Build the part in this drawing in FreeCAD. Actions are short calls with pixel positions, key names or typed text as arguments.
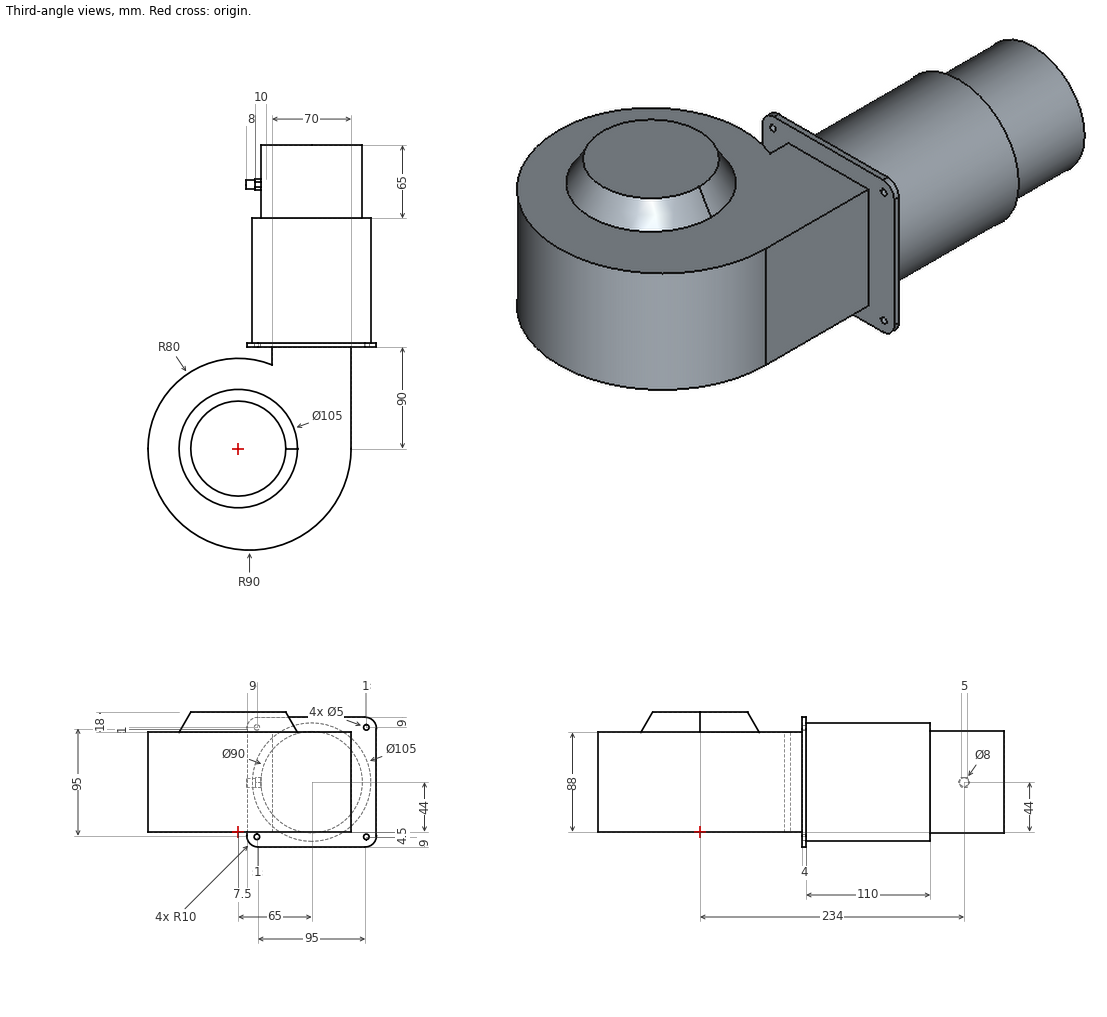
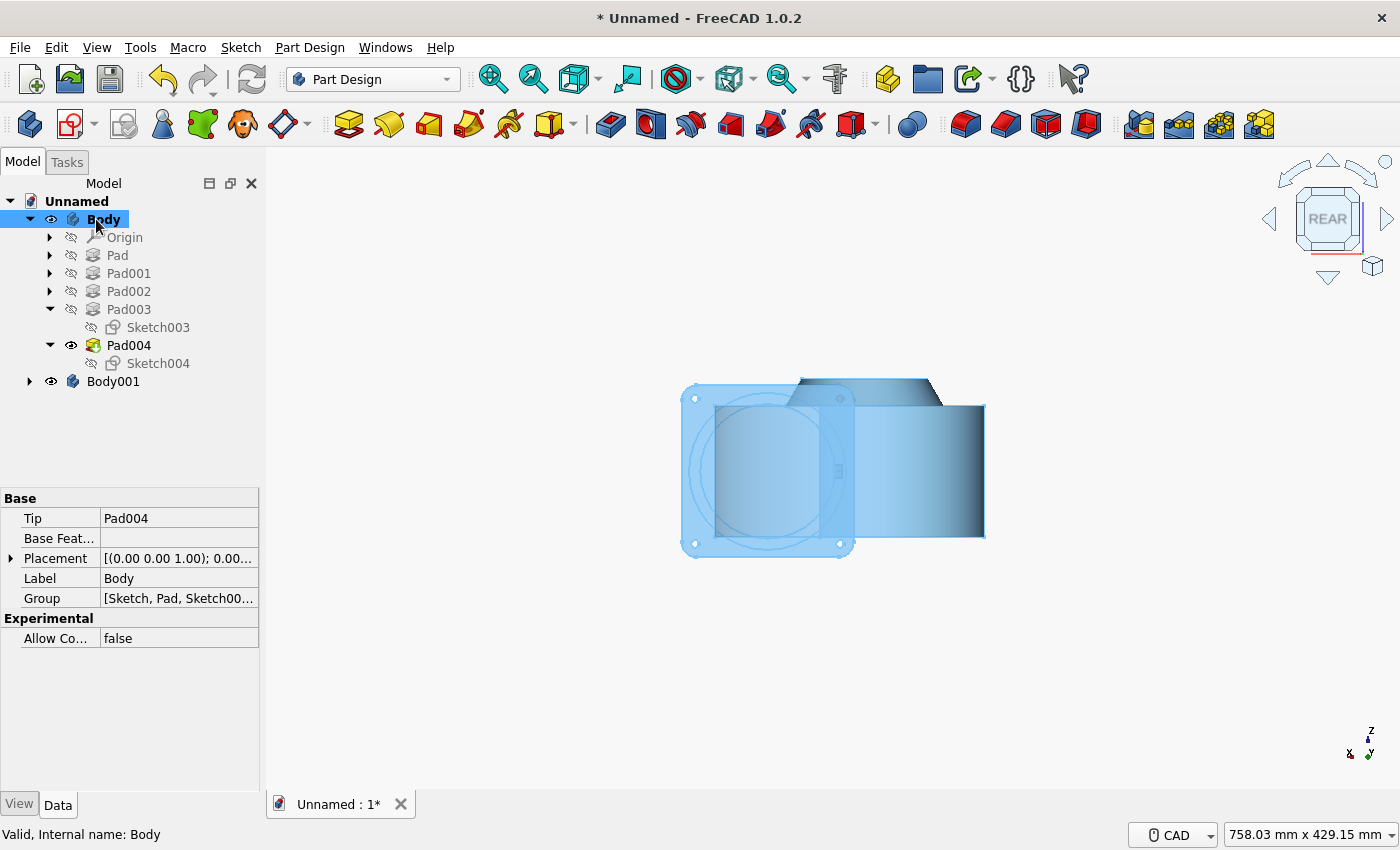
click(96, 381)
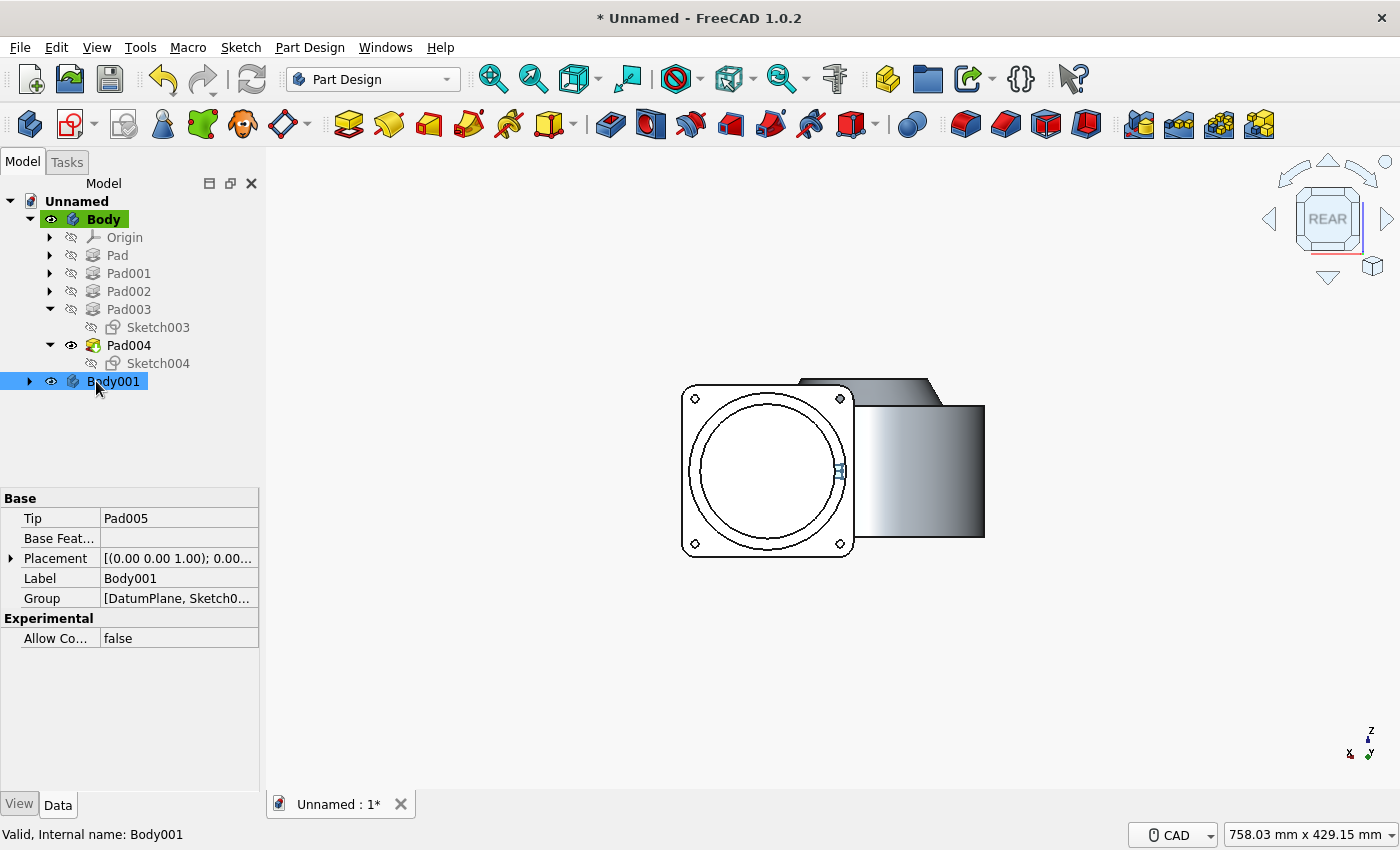
click(914, 124)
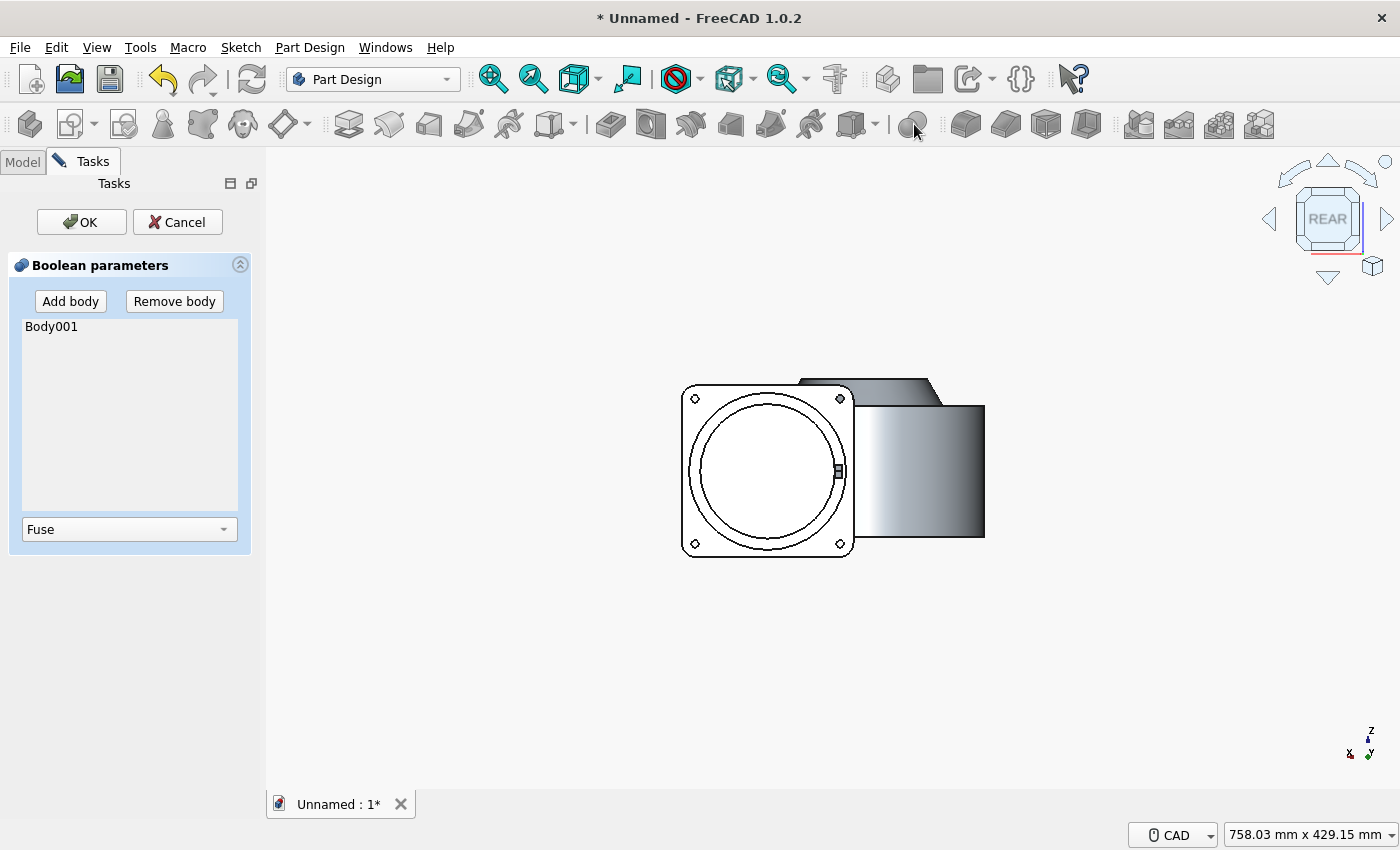
click(82, 222)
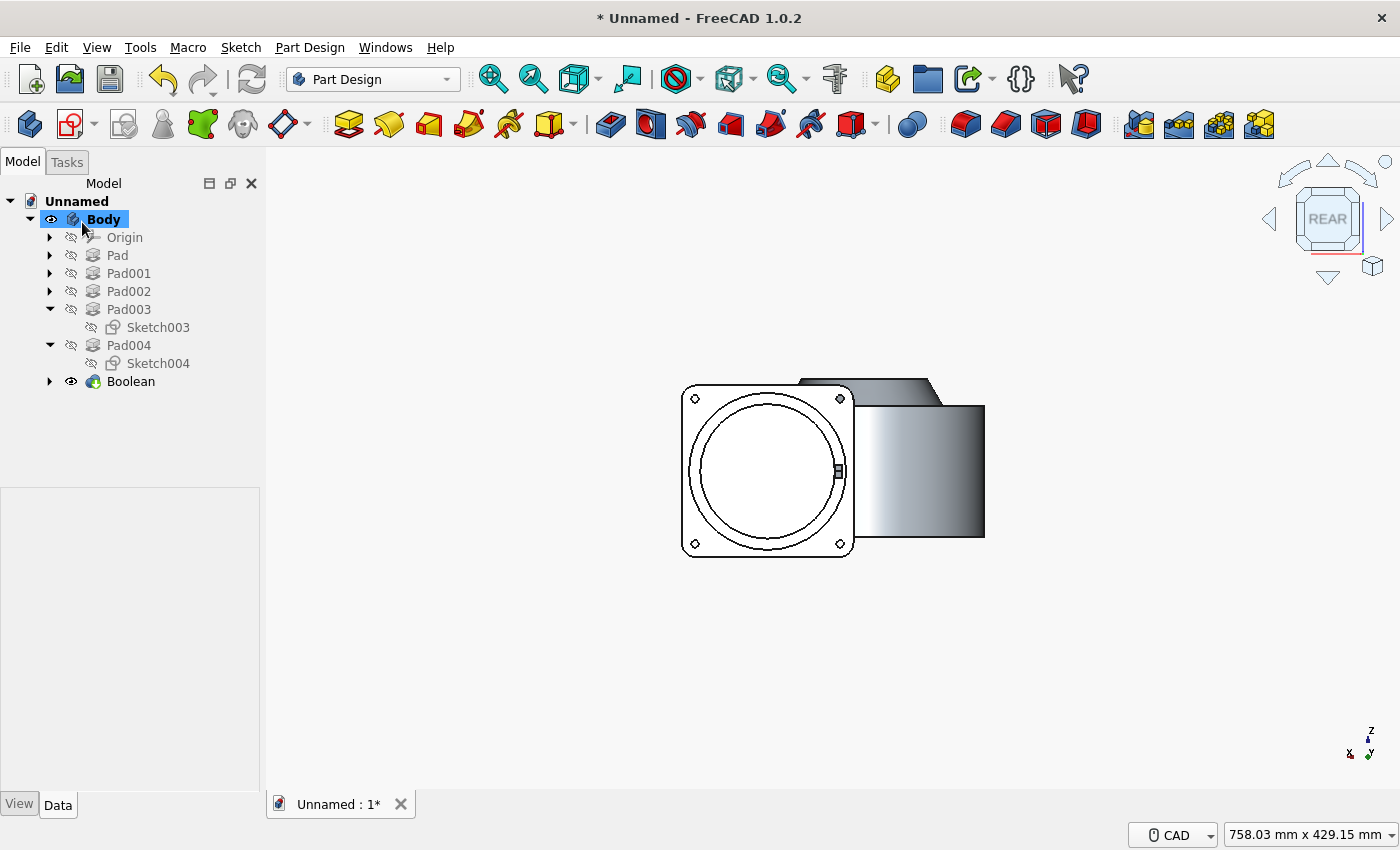
key(v)
key(f)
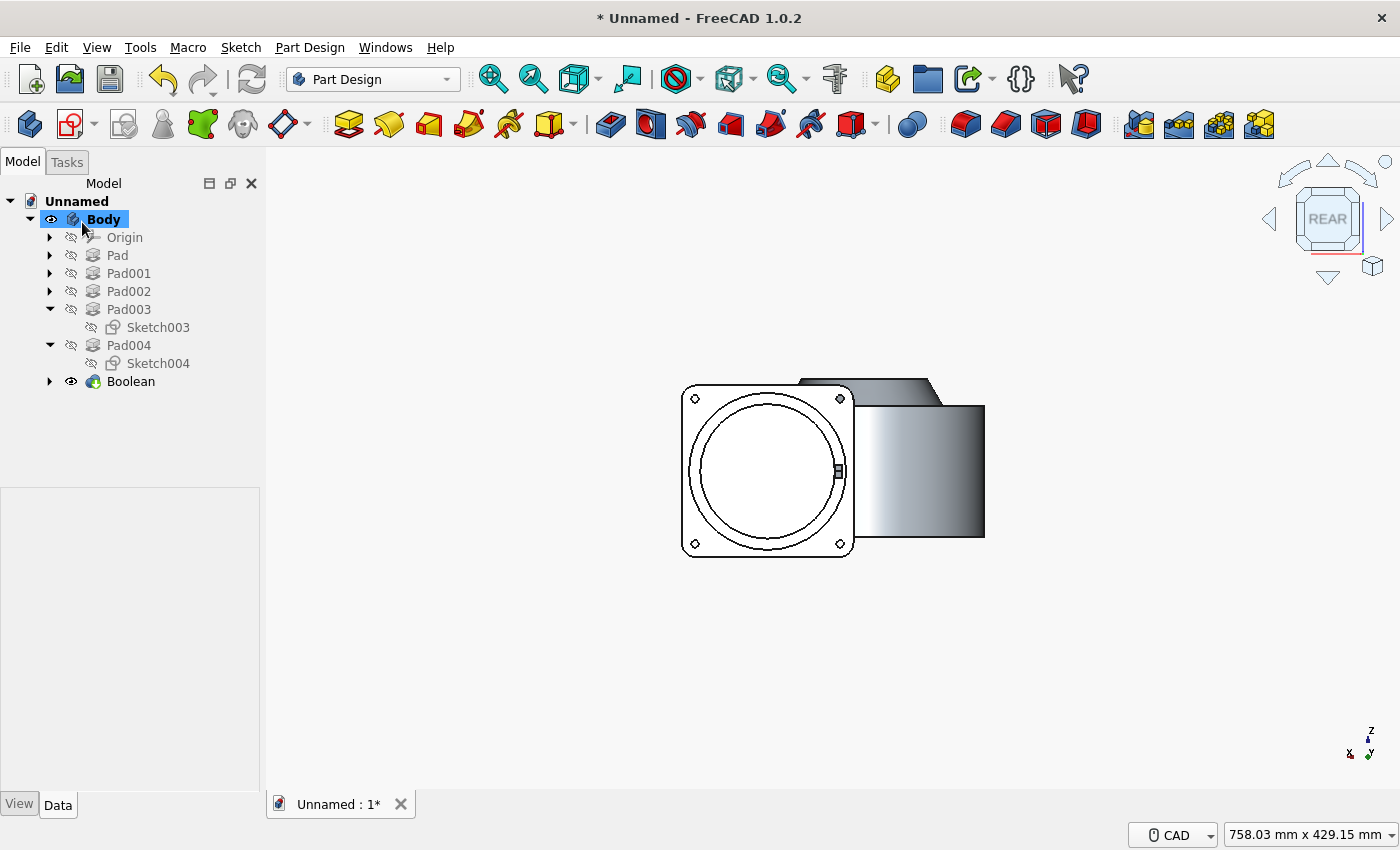
key(6)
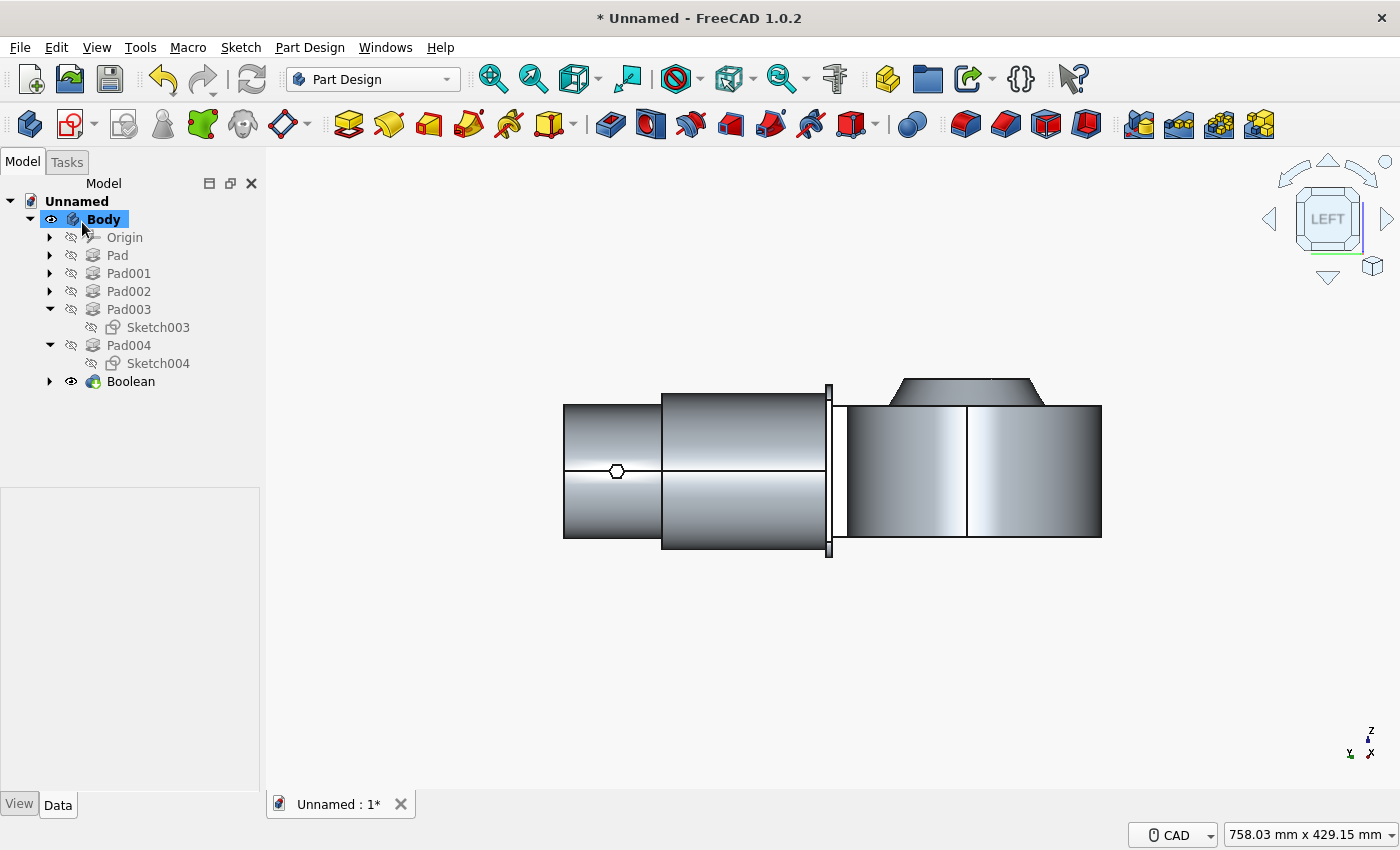
scroll(617, 470, up, 4)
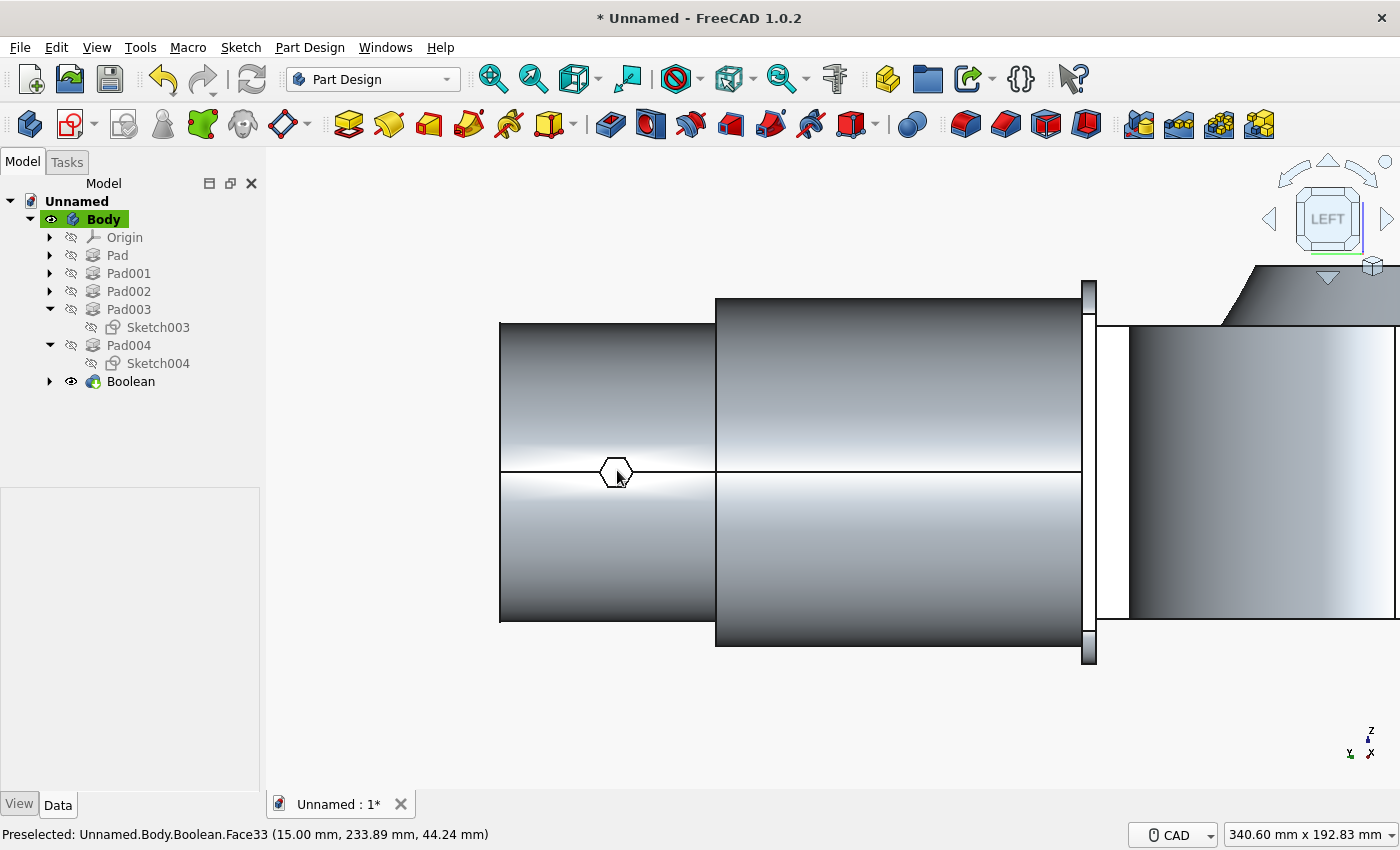
click(616, 471)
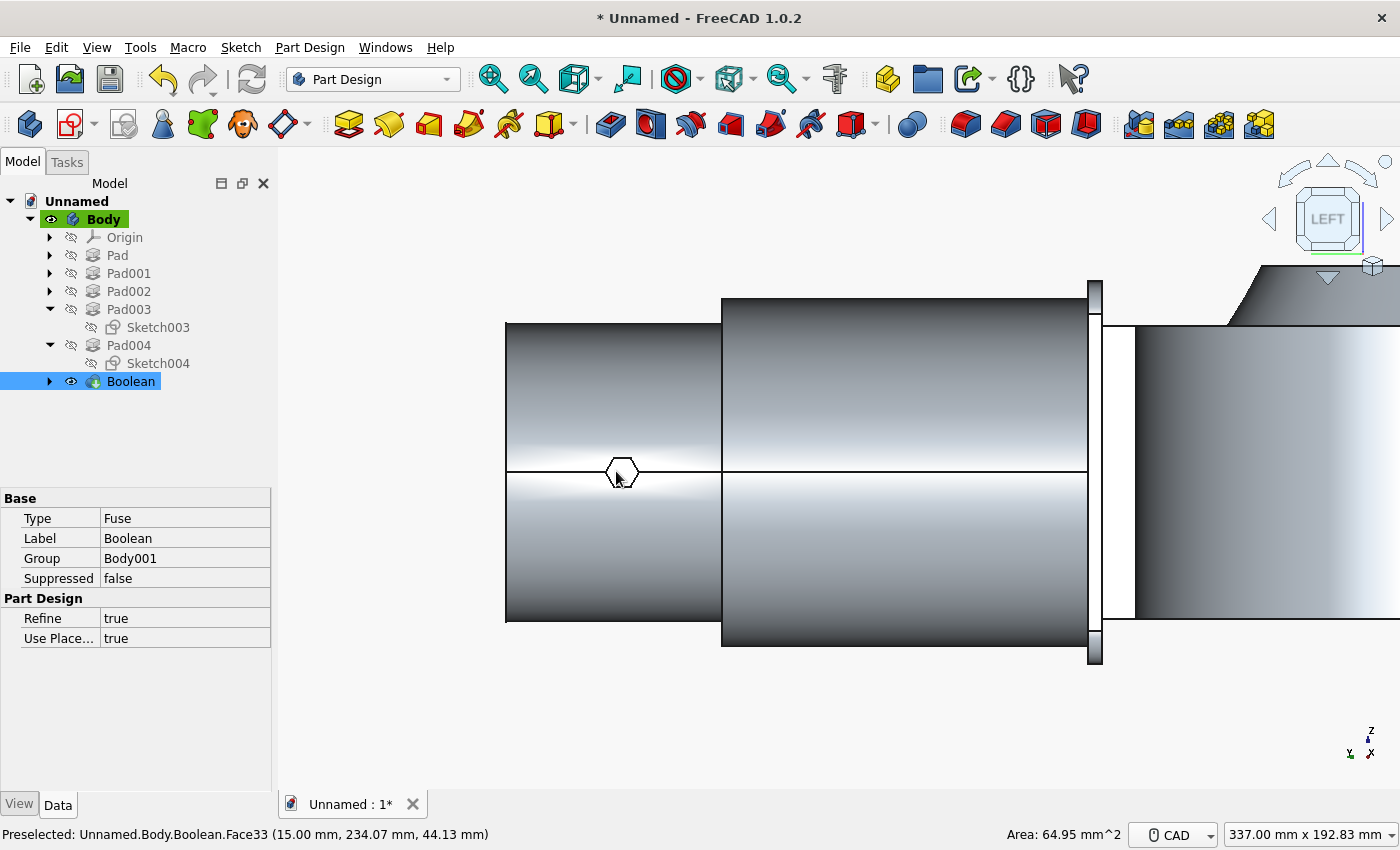
click(70, 124)